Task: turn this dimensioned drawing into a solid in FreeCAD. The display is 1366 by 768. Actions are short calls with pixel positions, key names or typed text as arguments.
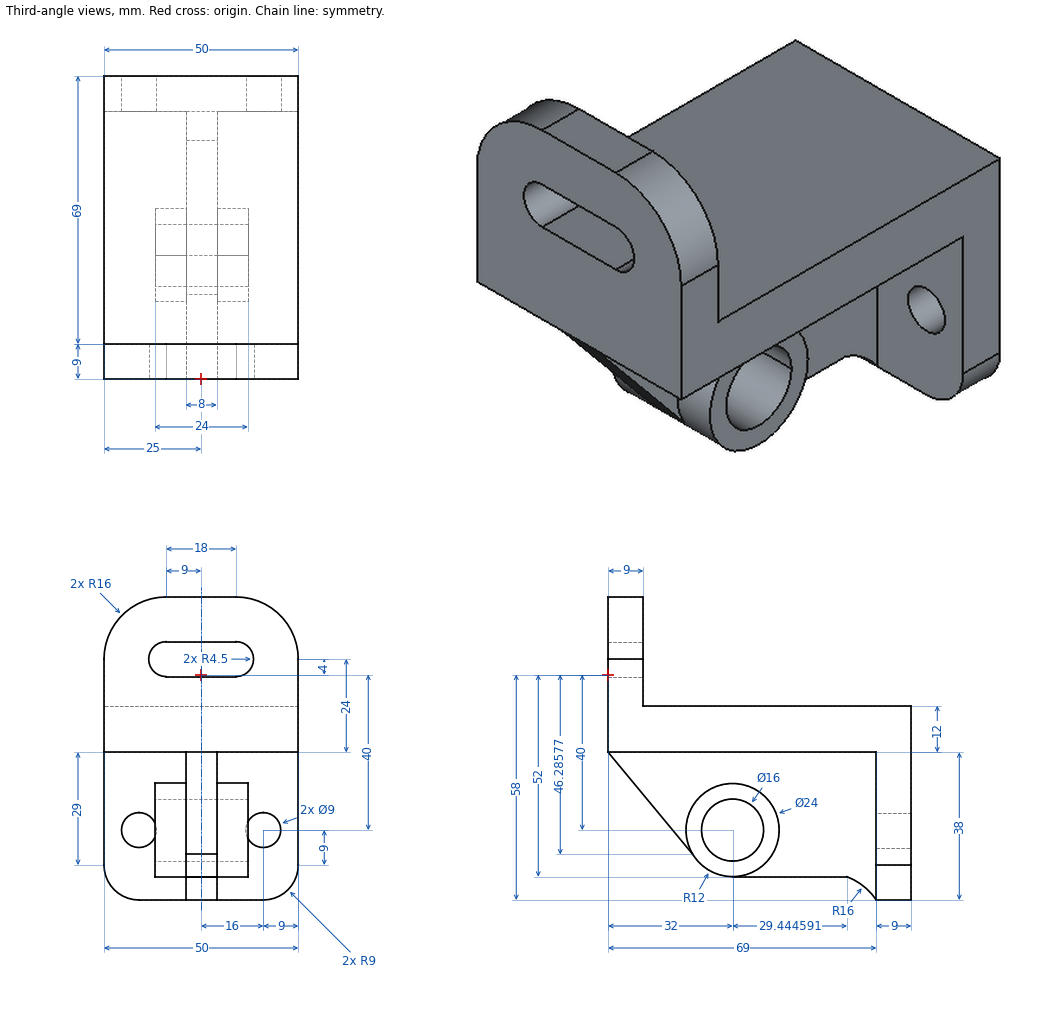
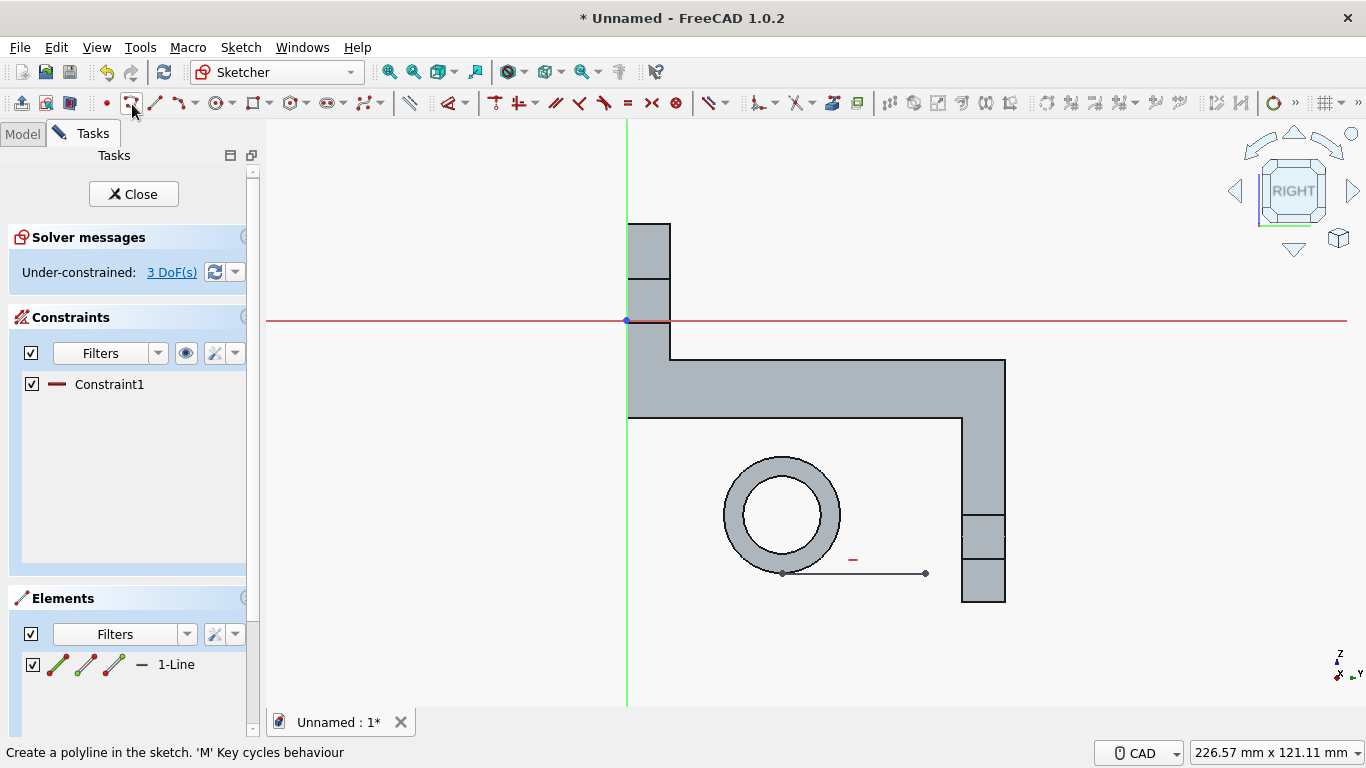
click(962, 602)
click(962, 418)
click(627, 418)
click(732, 545)
right_click(732, 545)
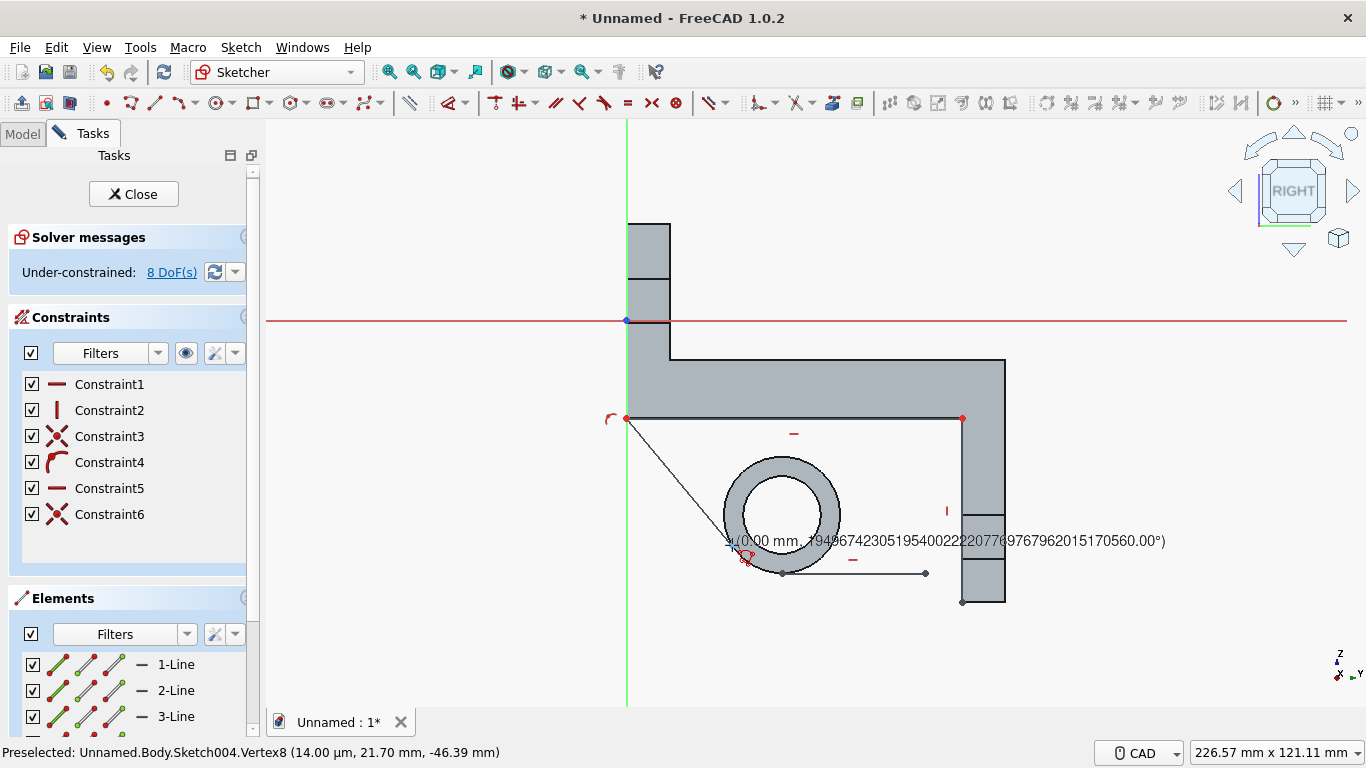
click(180, 104)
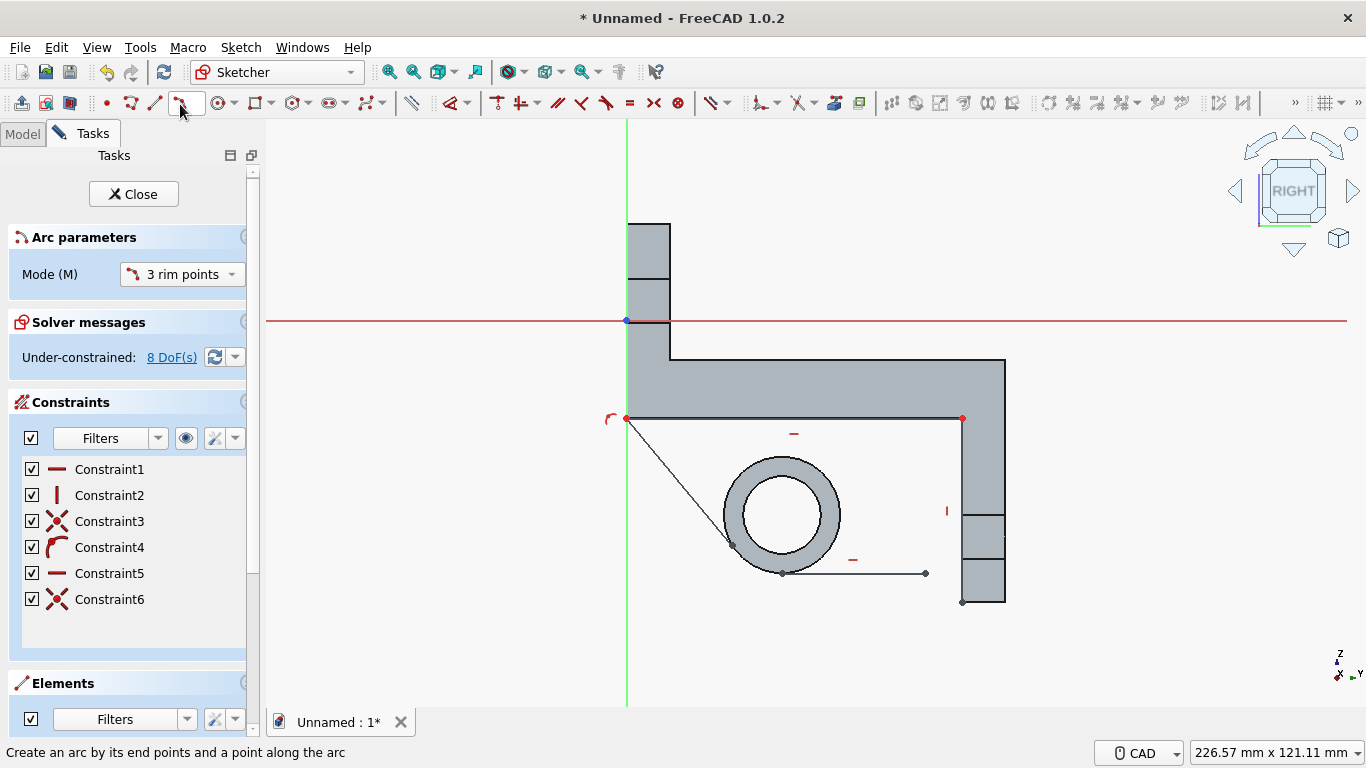
click(925, 574)
click(962, 603)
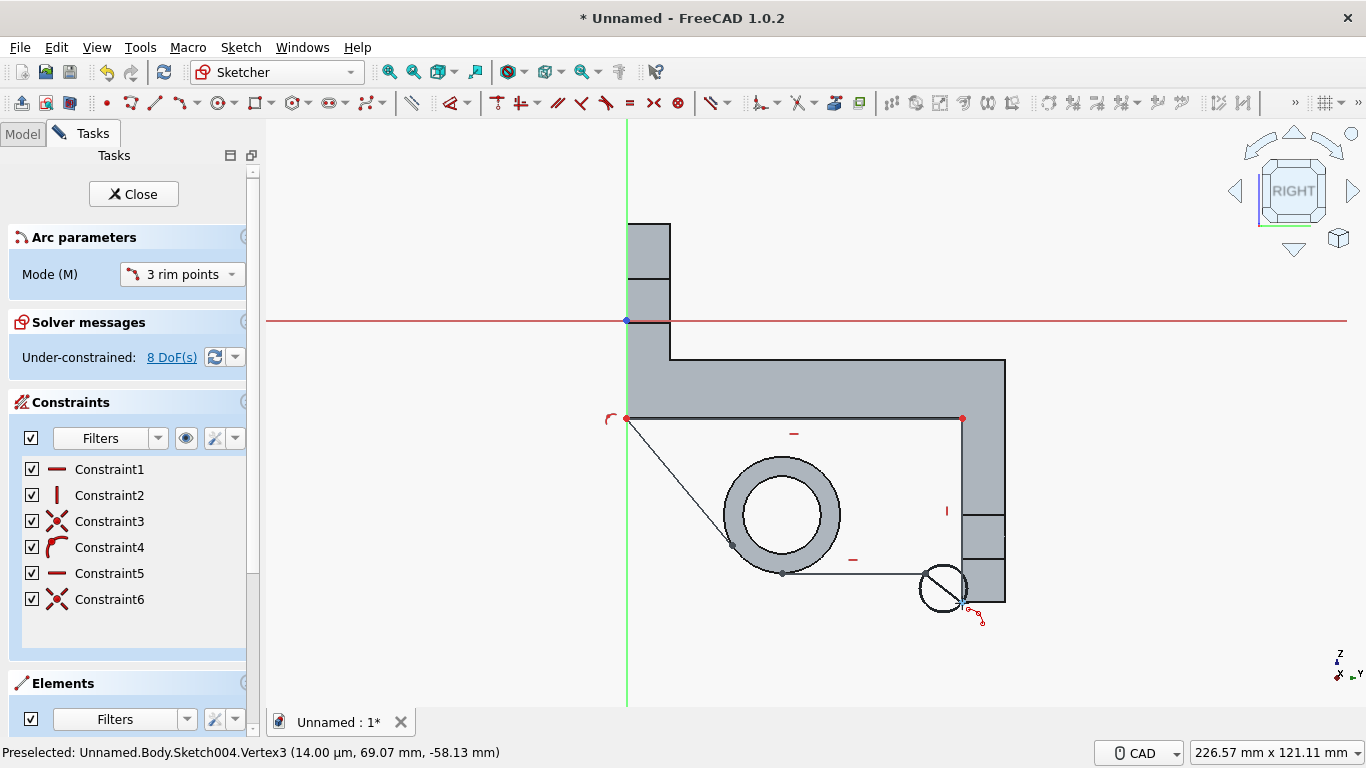
scroll(946, 585, up, 8)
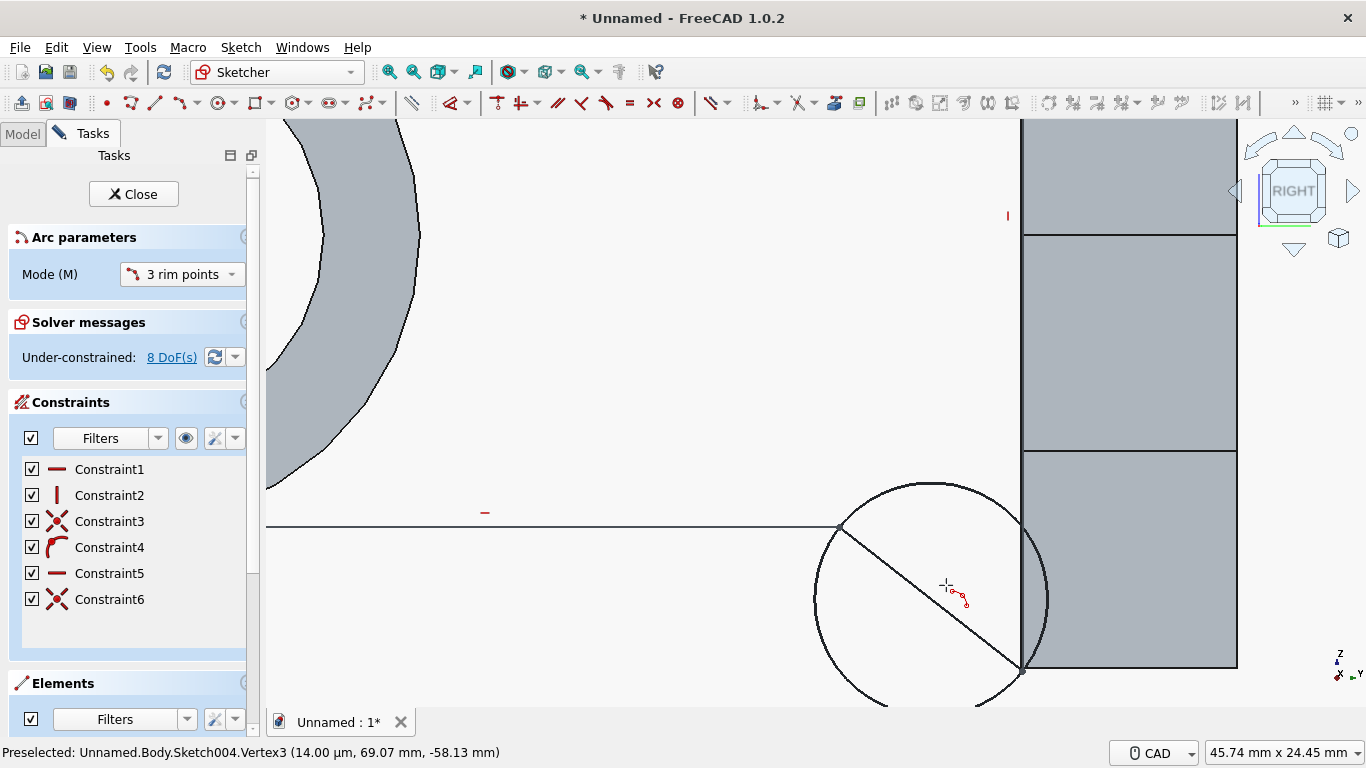
click(941, 582)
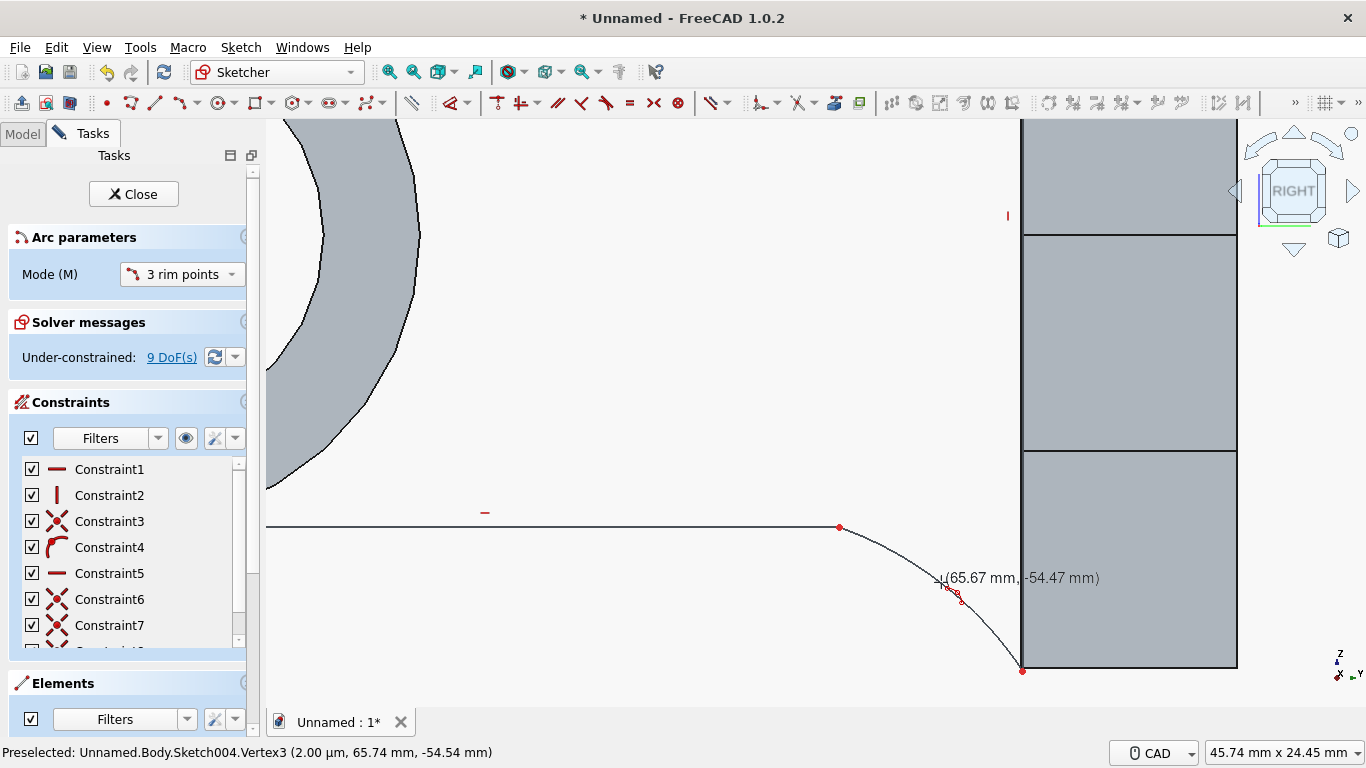
scroll(930, 558, down, 7)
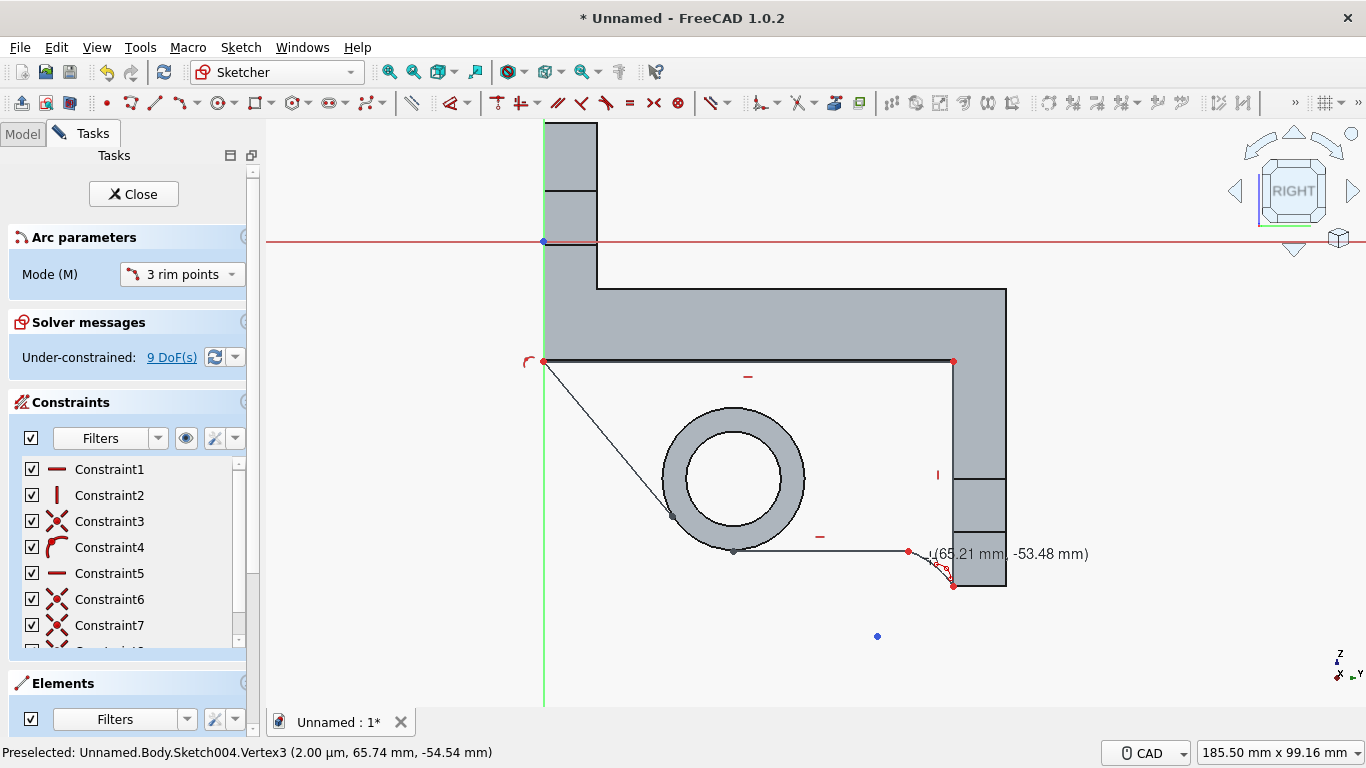
click(672, 517)
click(733, 551)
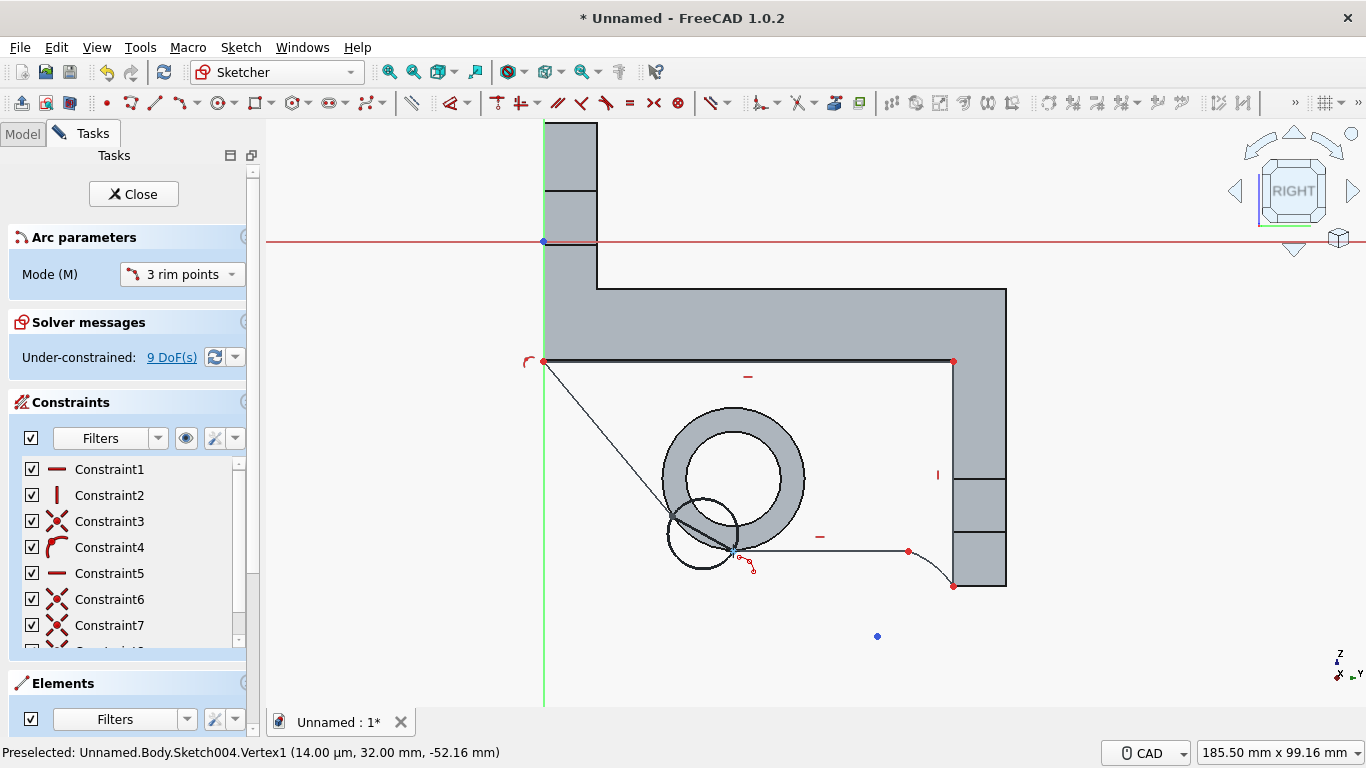
scroll(699, 541, up, 3)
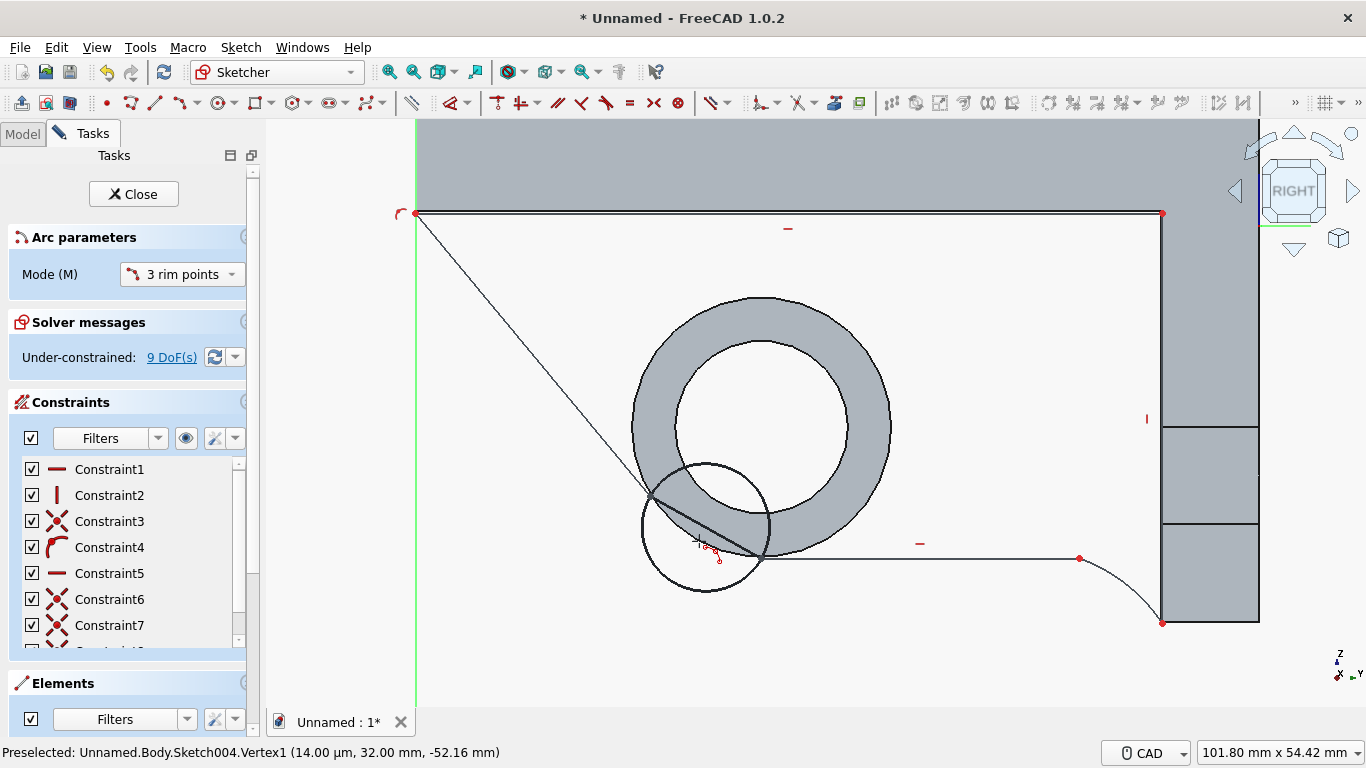
click(698, 540)
key(Escape)